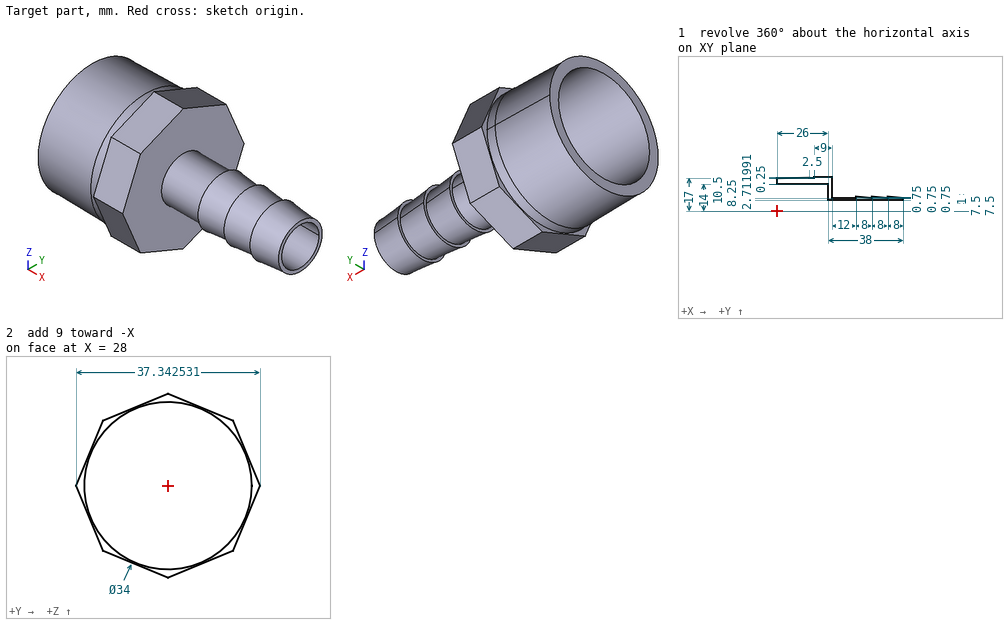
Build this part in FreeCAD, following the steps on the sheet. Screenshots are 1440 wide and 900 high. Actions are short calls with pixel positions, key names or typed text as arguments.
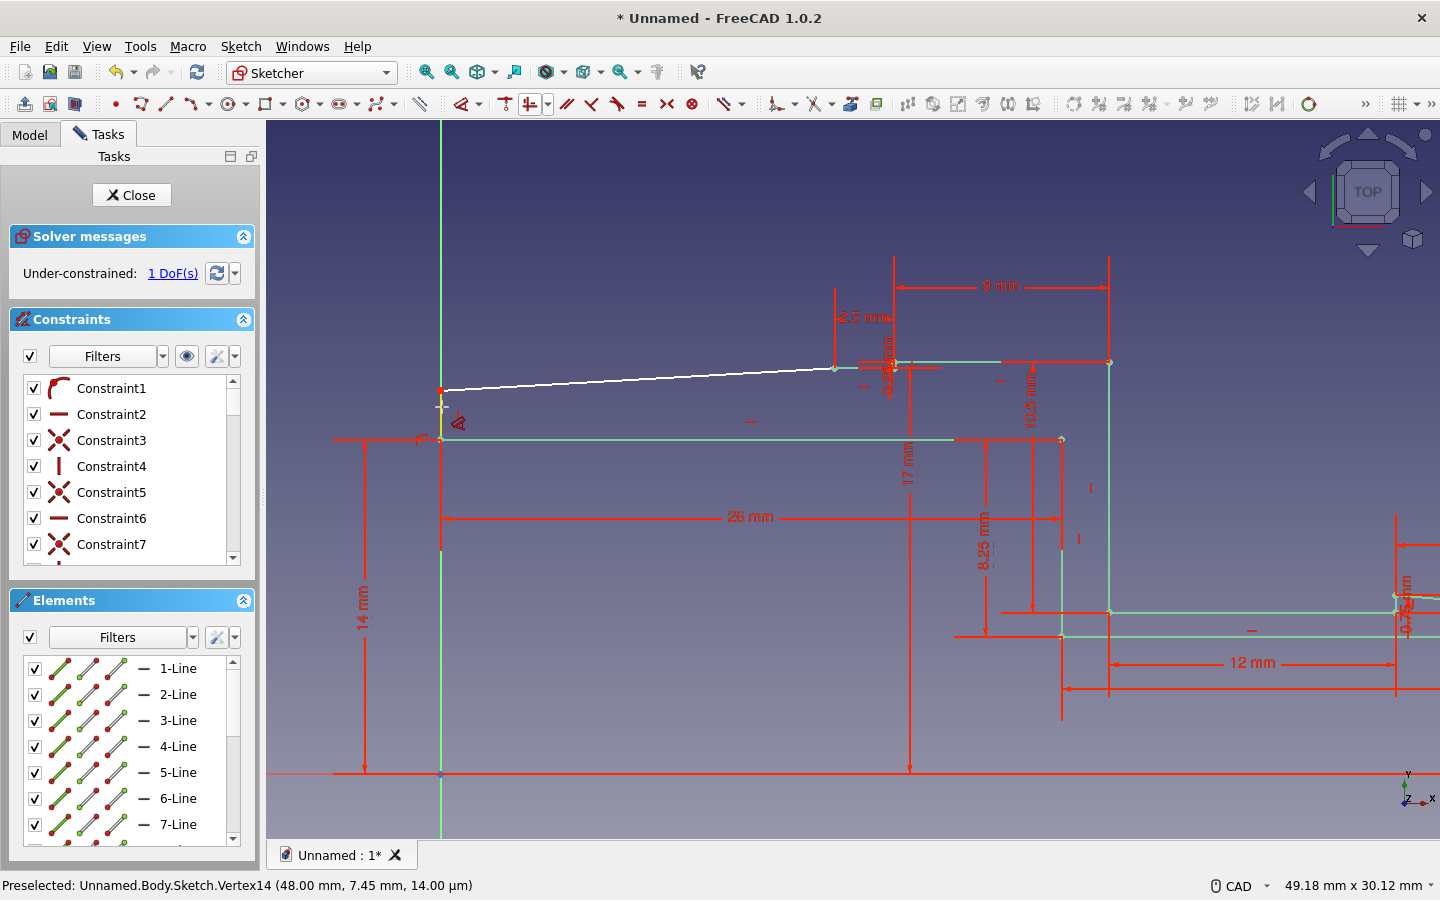
click(441, 406)
click(407, 415)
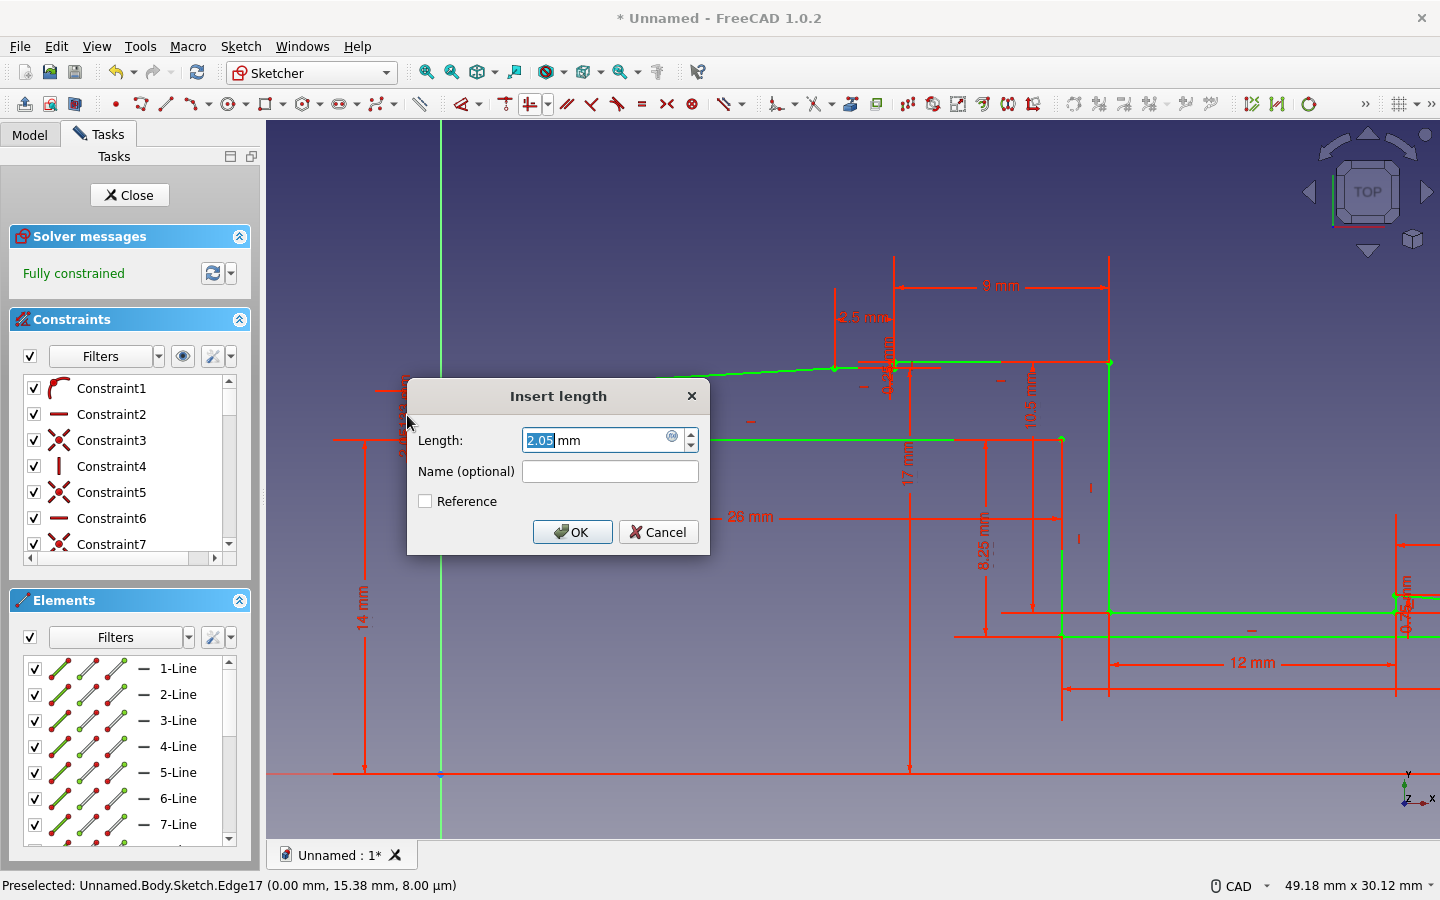
text(2.711991)
key(Return)
key(Escape)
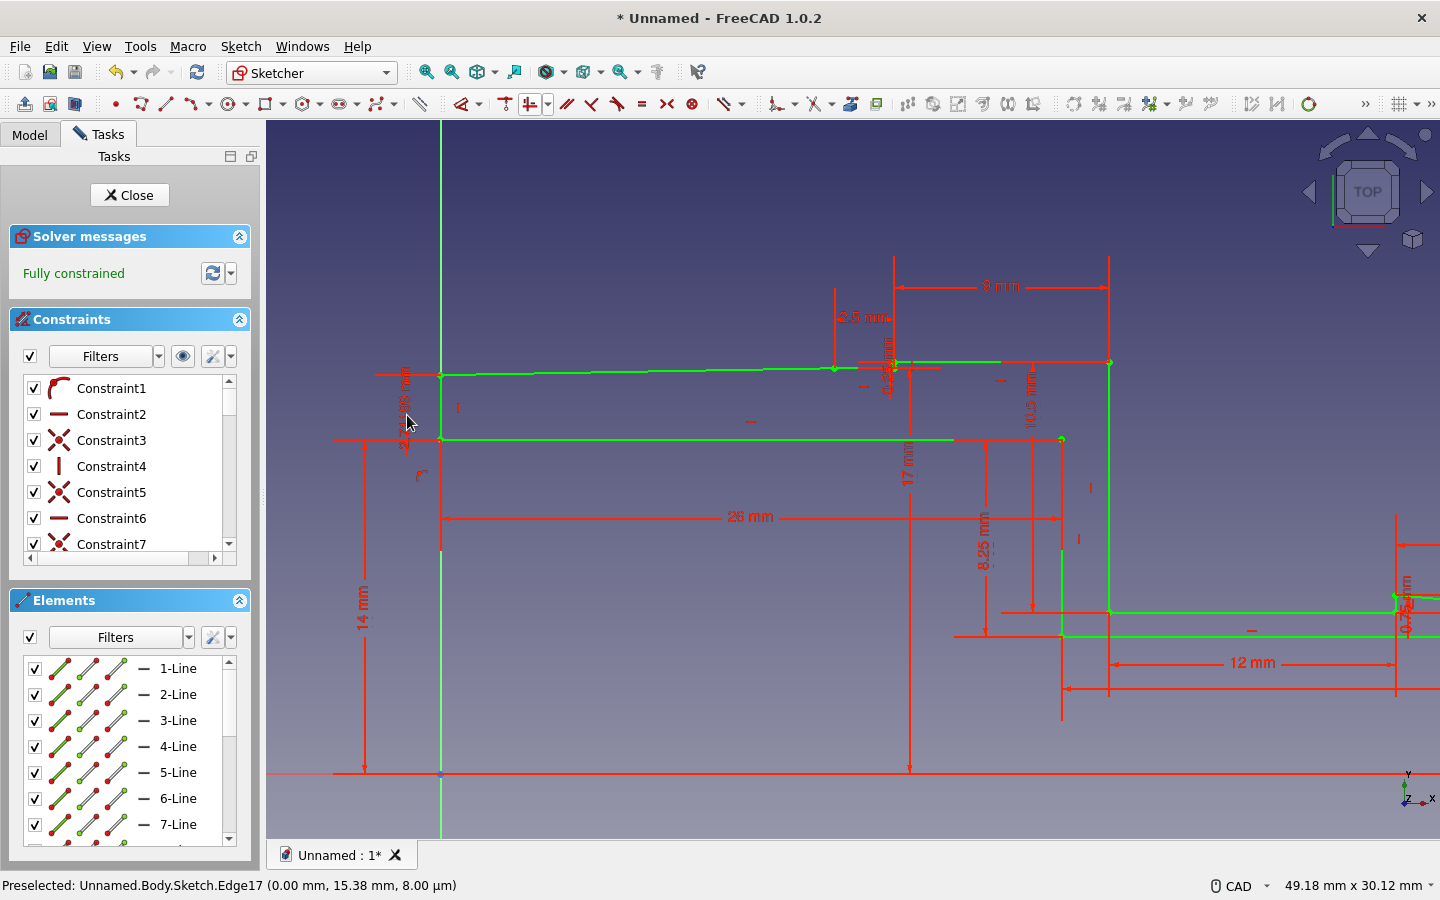
click(130, 195)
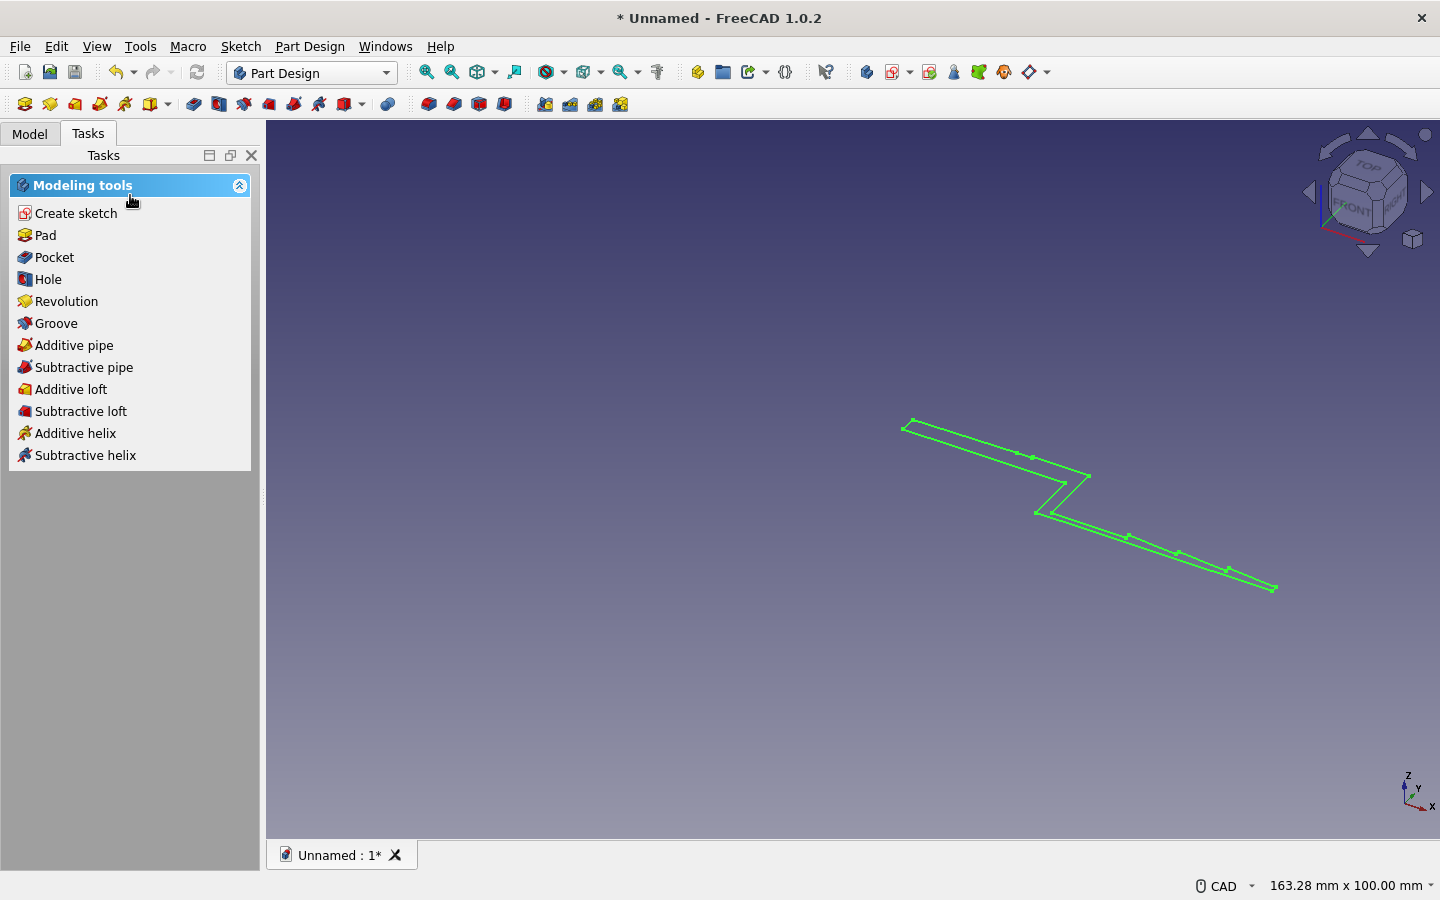
click(50, 104)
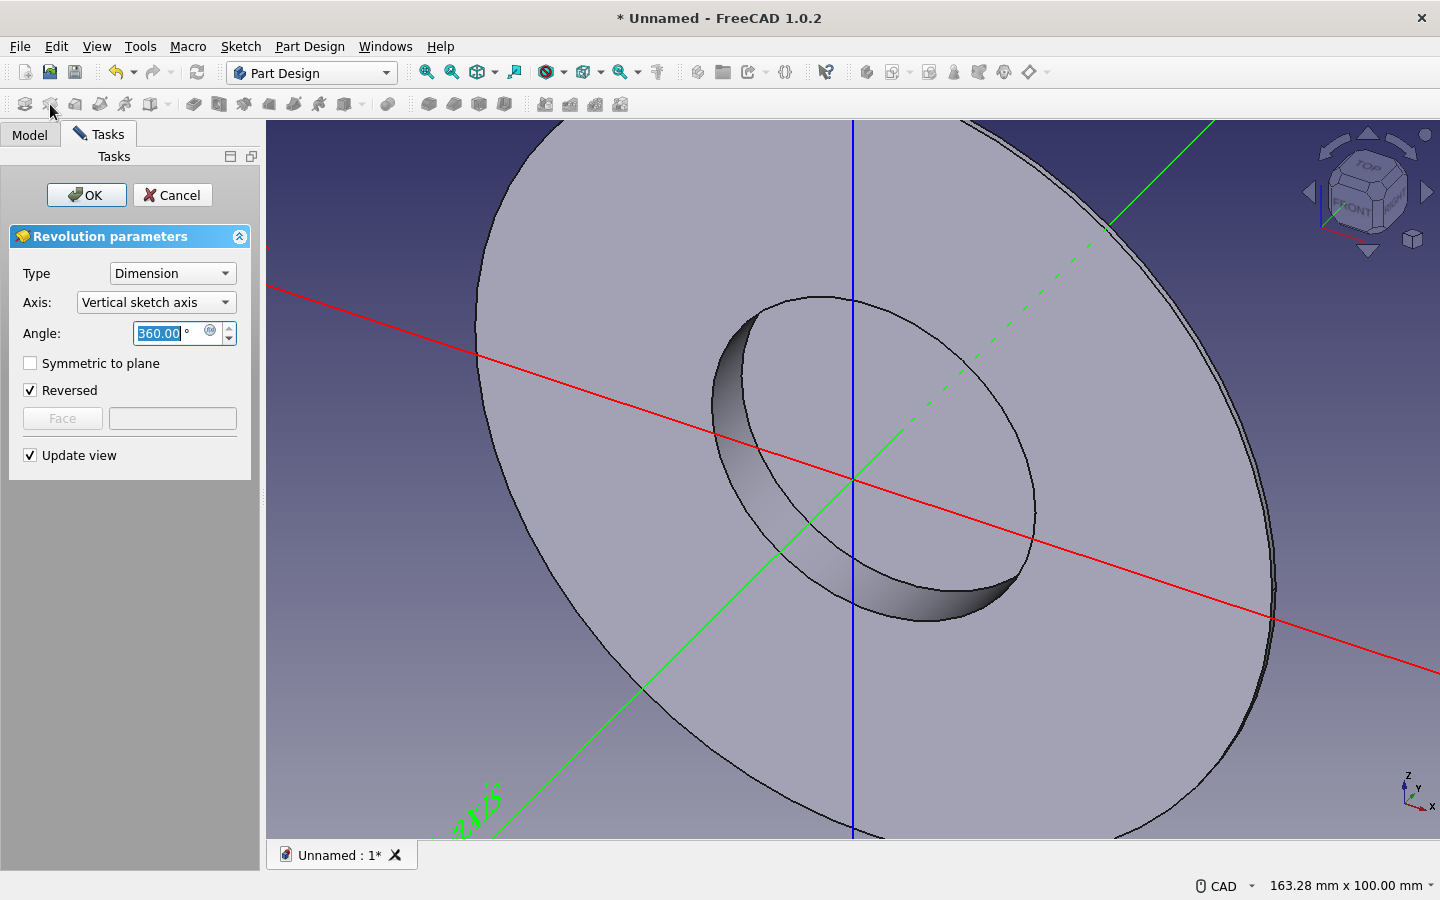
click(157, 302)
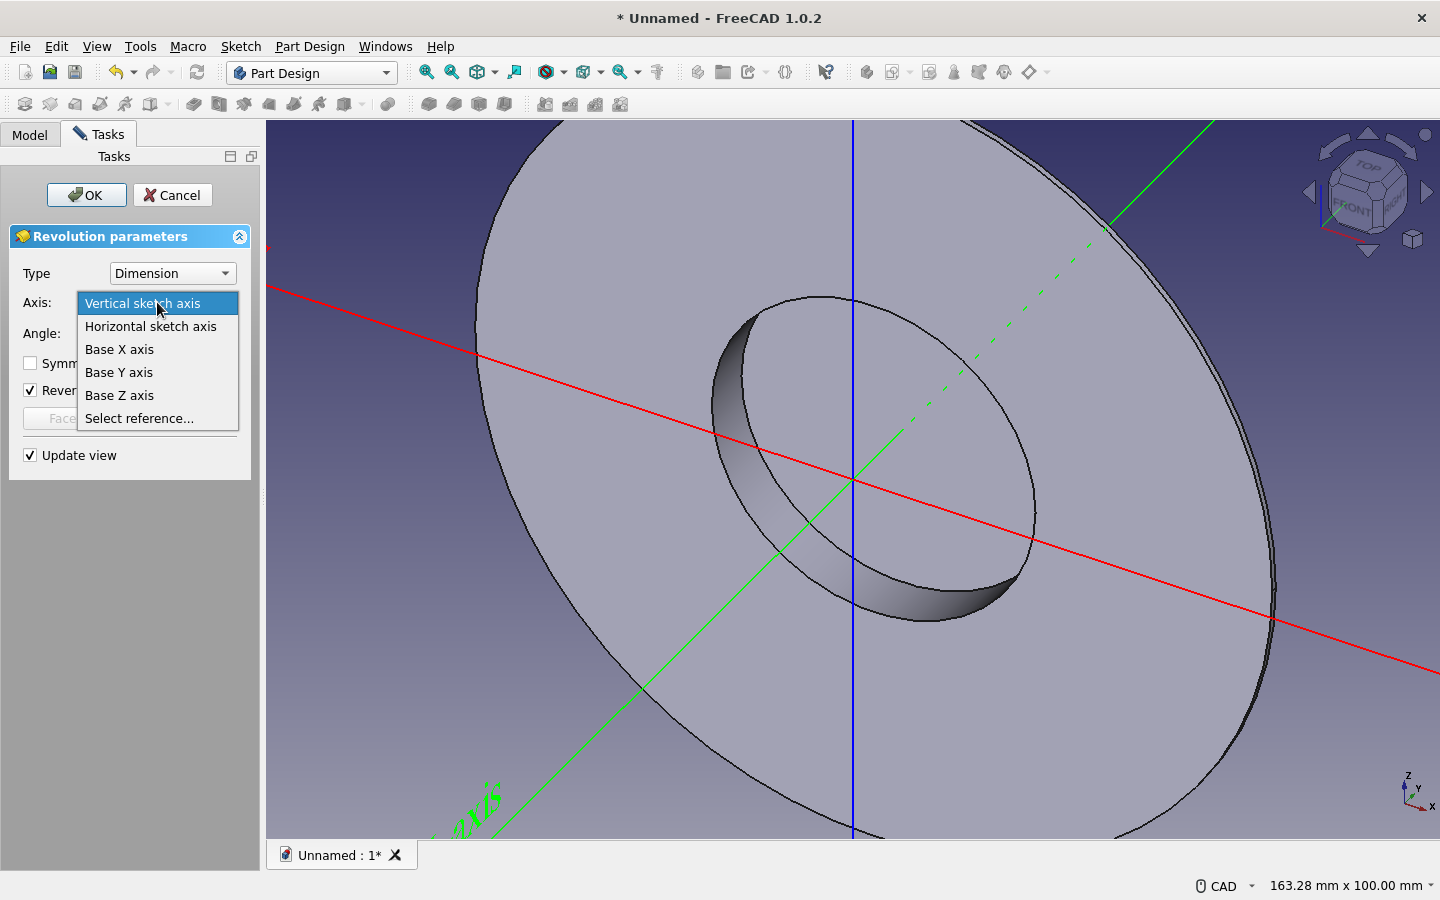
click(156, 326)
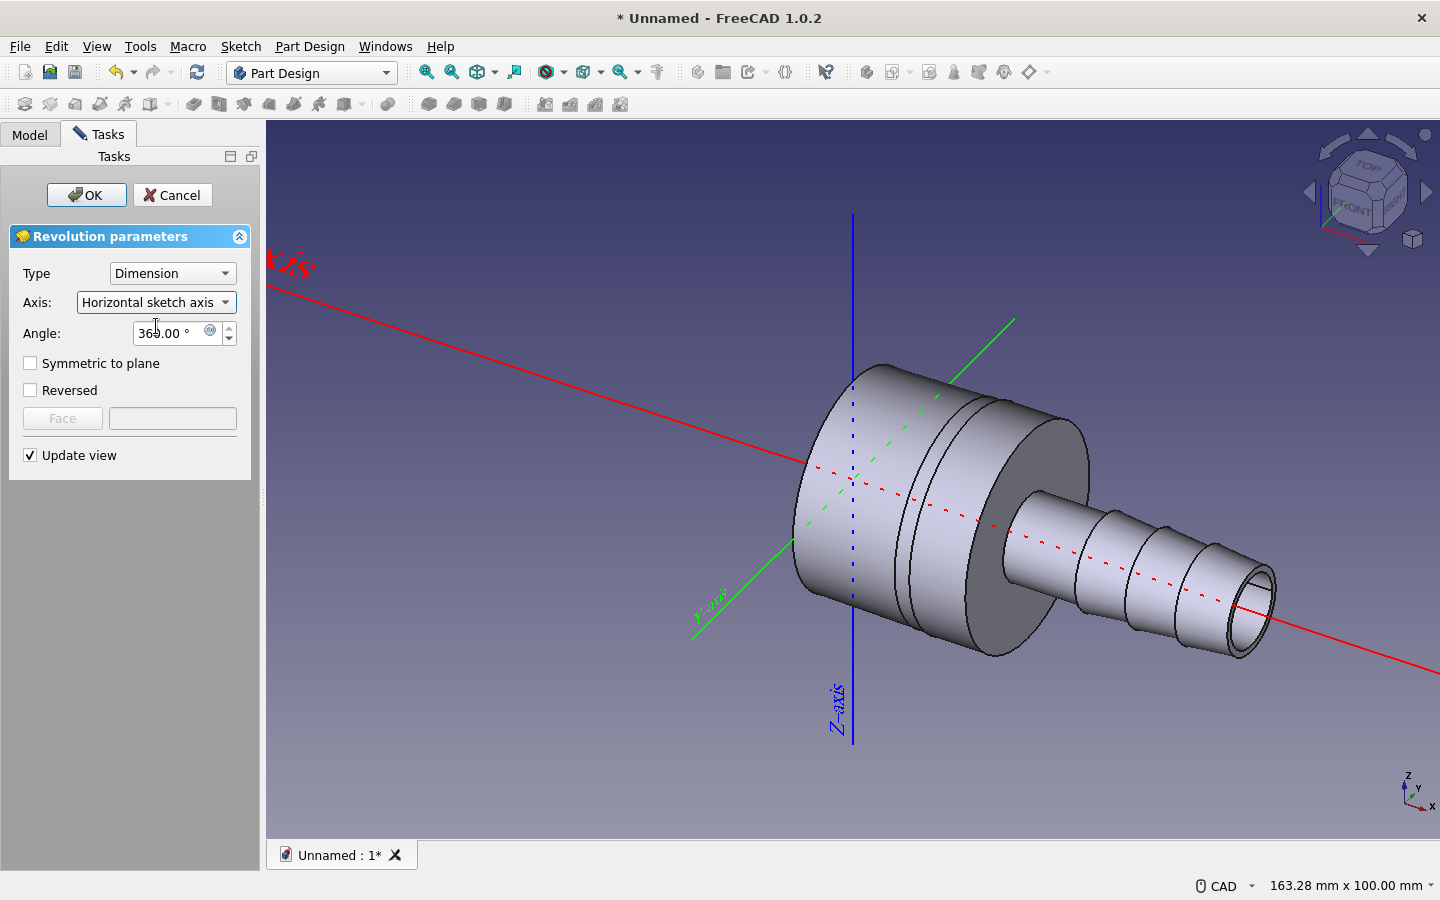
click(87, 195)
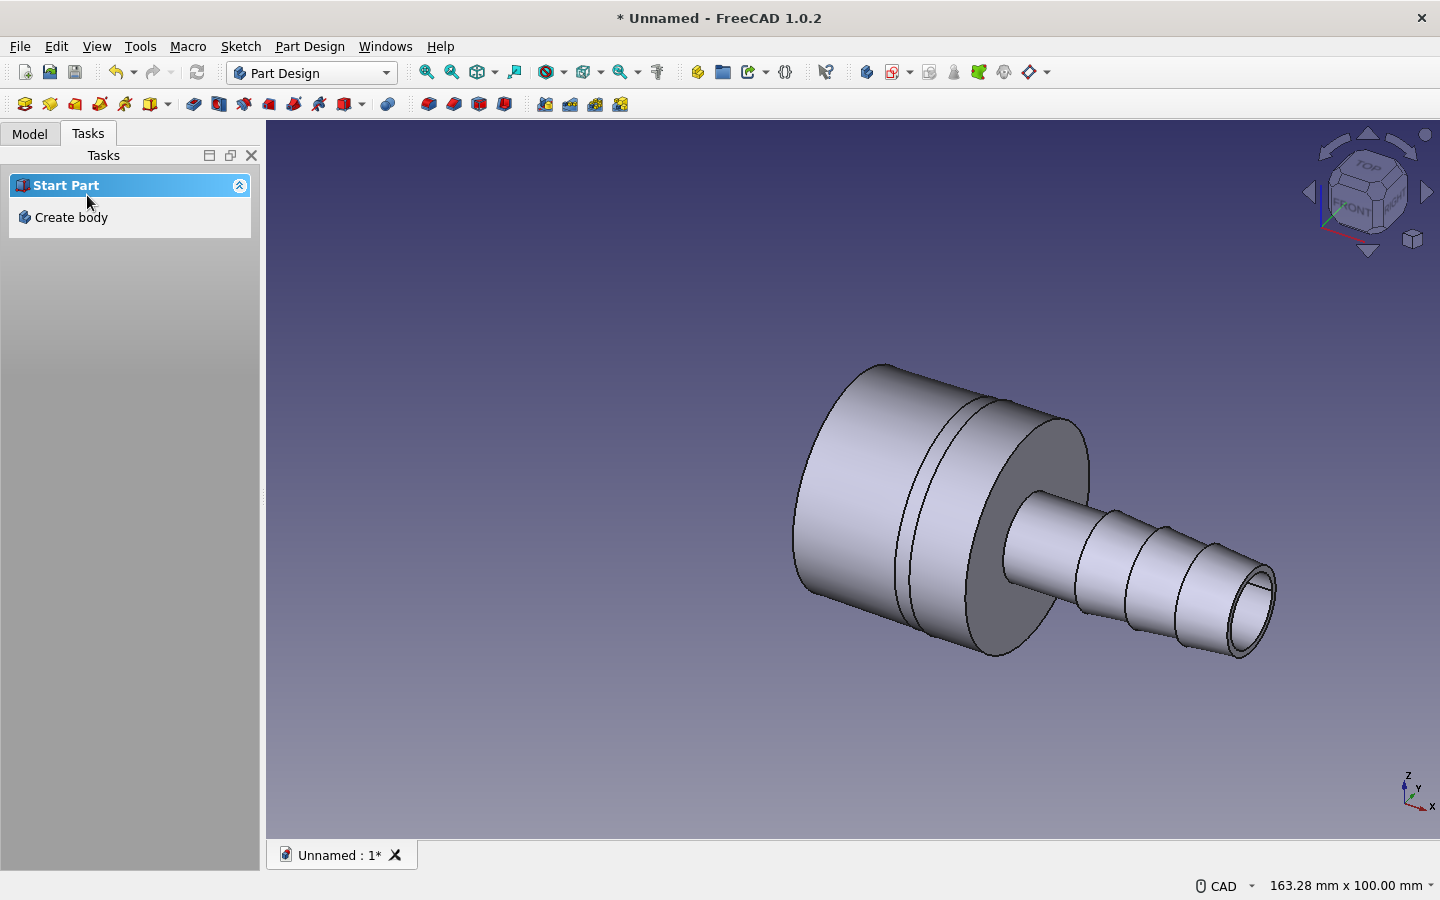
click(1045, 461)